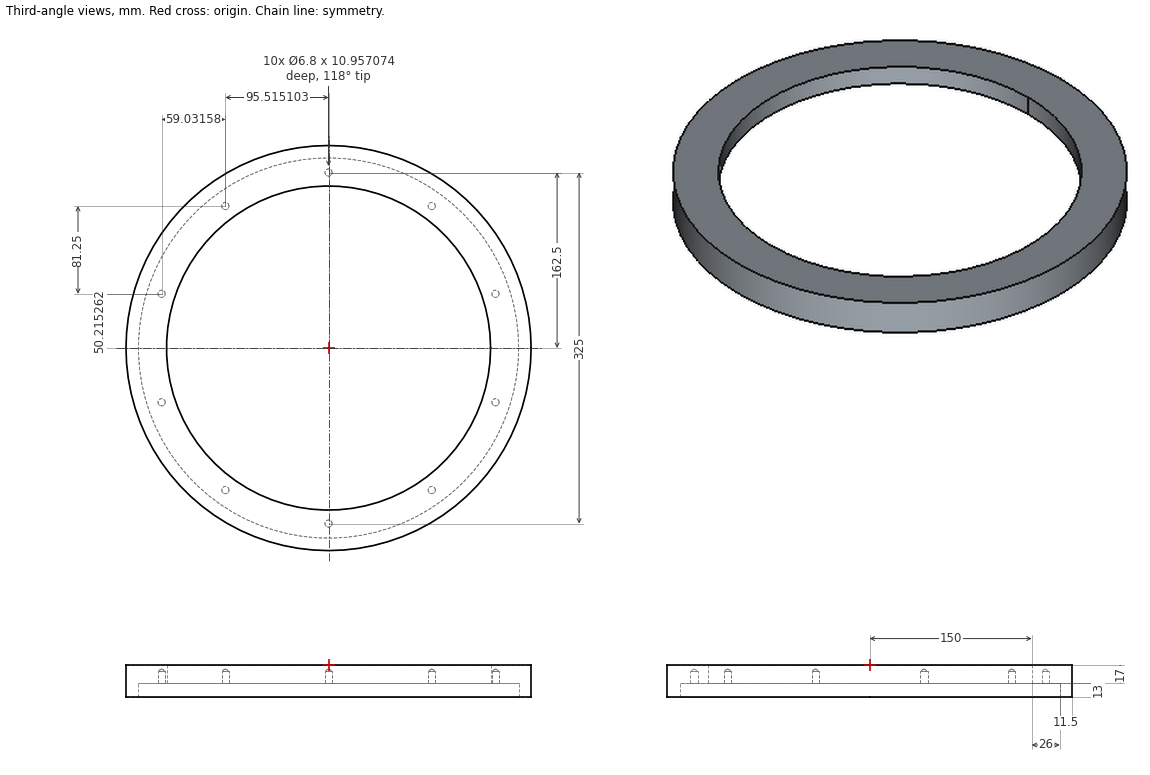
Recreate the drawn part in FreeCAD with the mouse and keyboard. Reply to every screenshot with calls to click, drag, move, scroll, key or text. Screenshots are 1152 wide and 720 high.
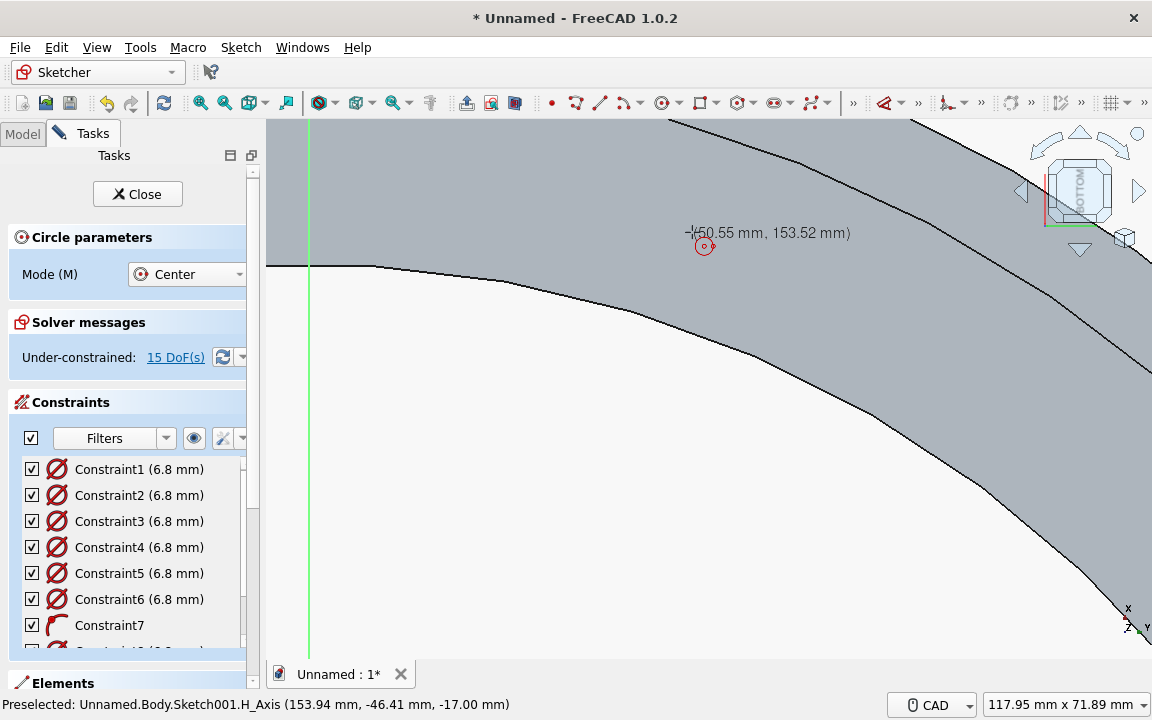
scroll(692, 232, down, 10)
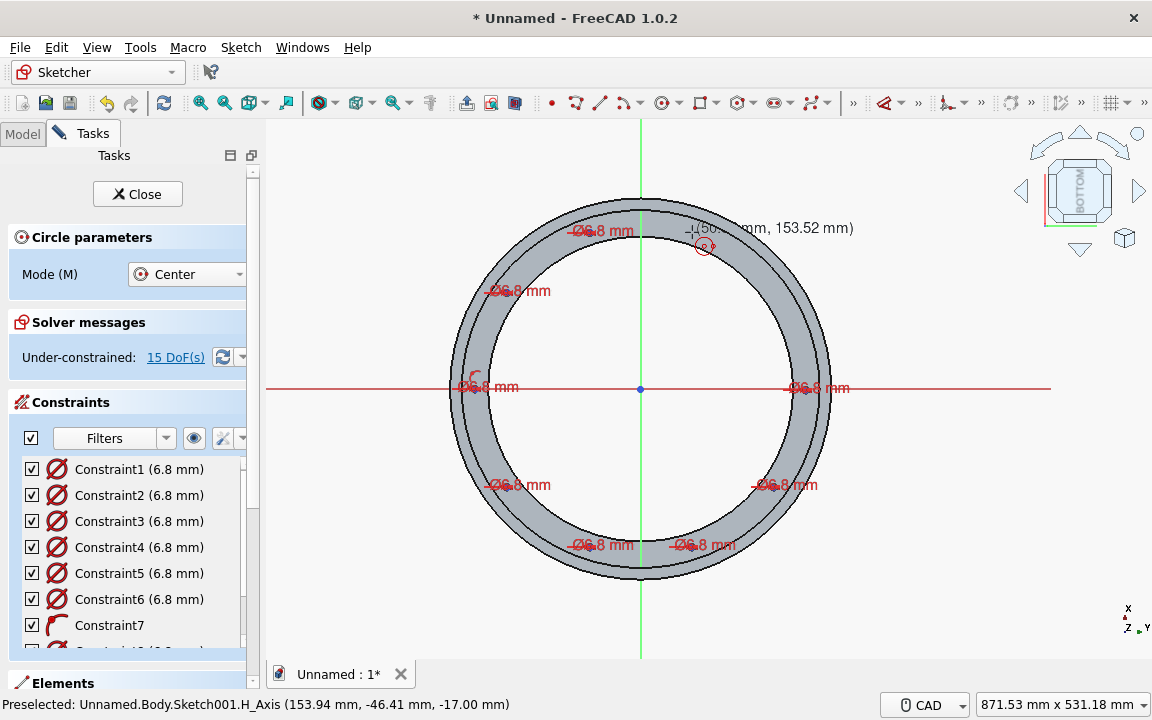
click(692, 232)
move(694, 230)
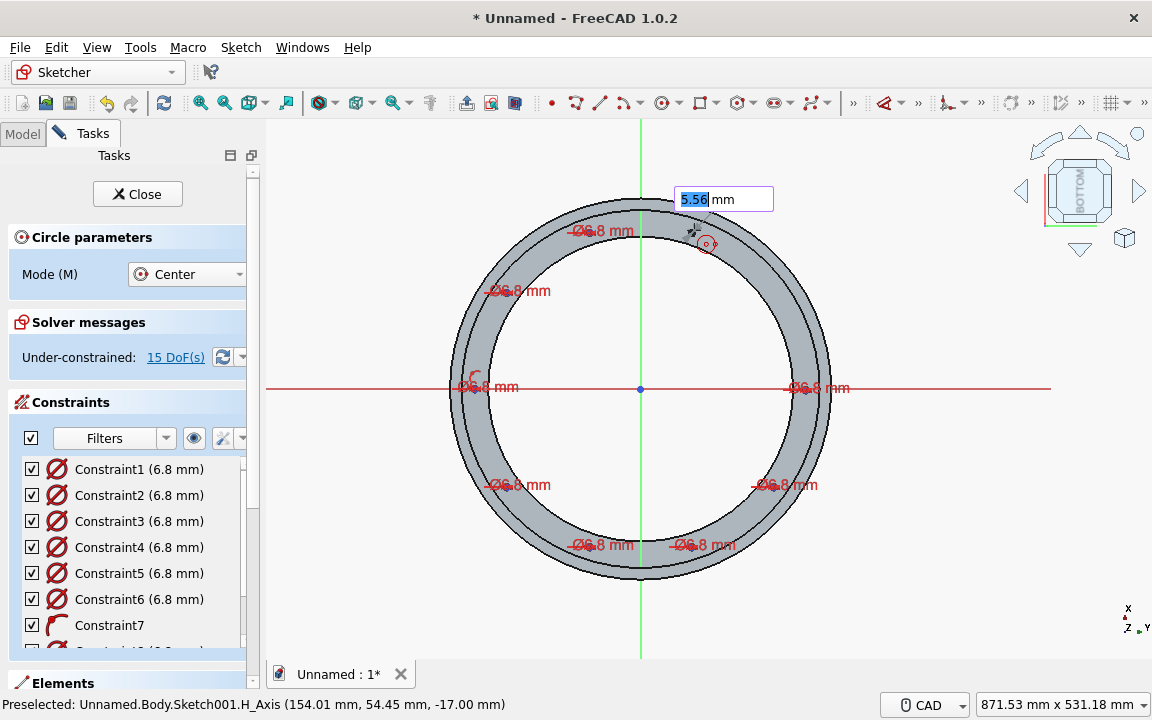
text(6.8)
key(Return)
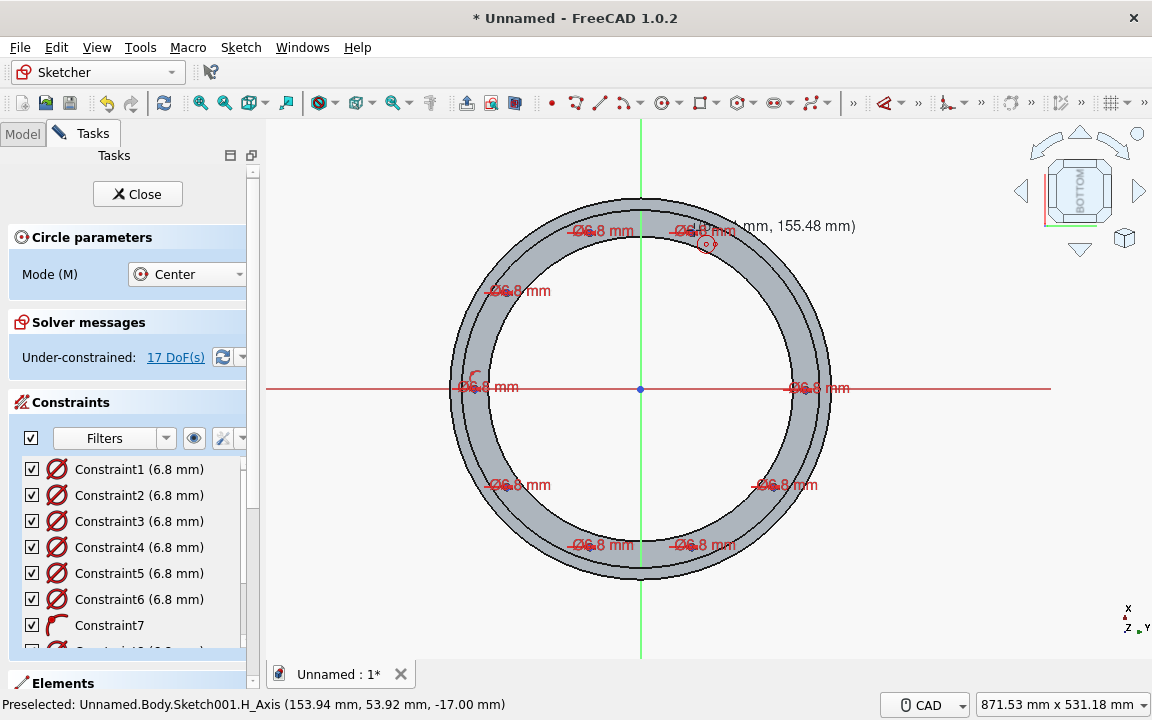
scroll(774, 292, up, 10)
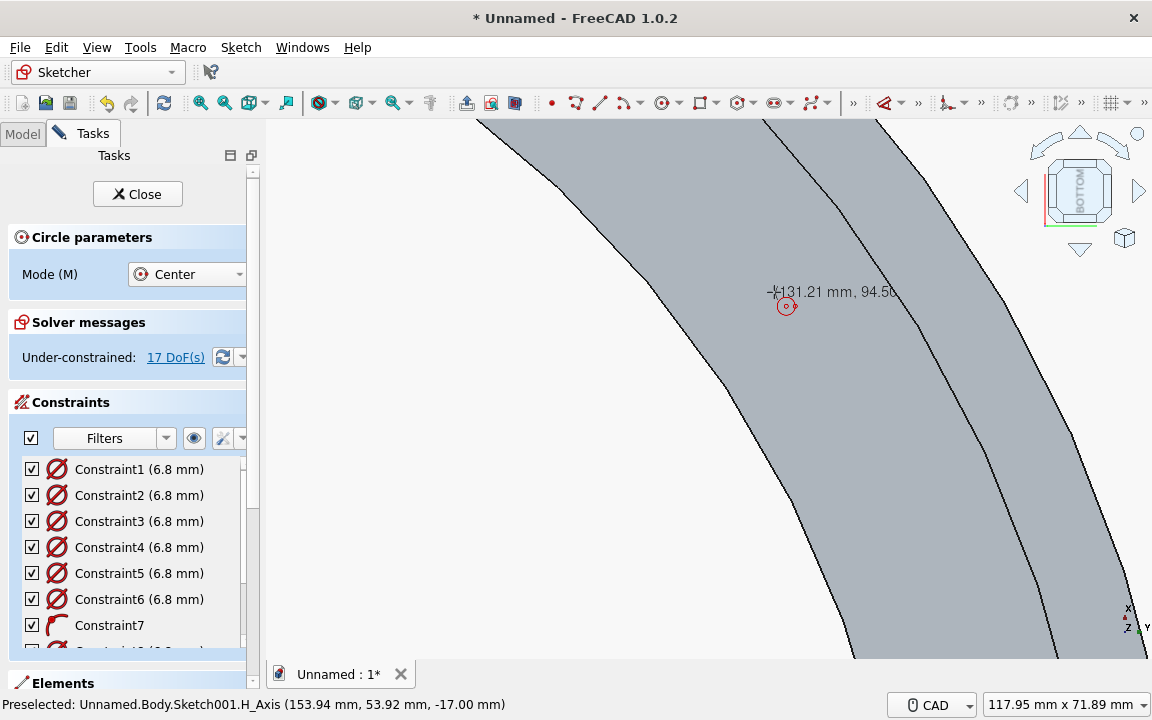
scroll(774, 292, down, 10)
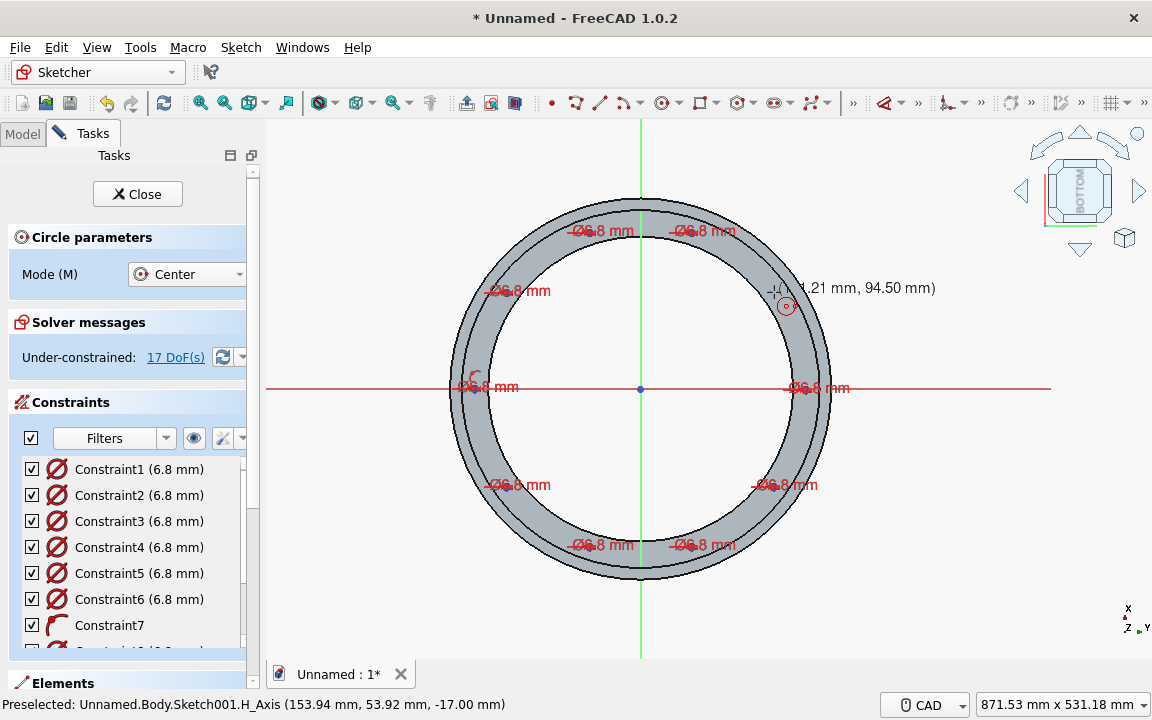
click(774, 292)
move(777, 290)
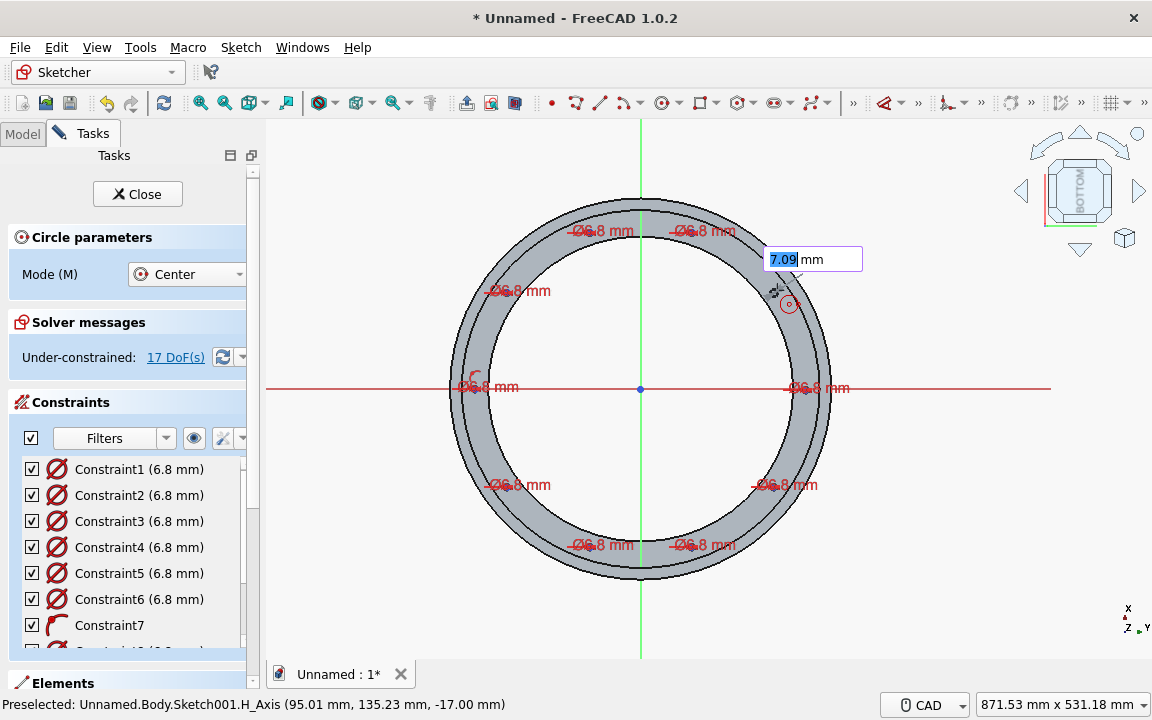
text(6.8)
key(Return)
key(Escape)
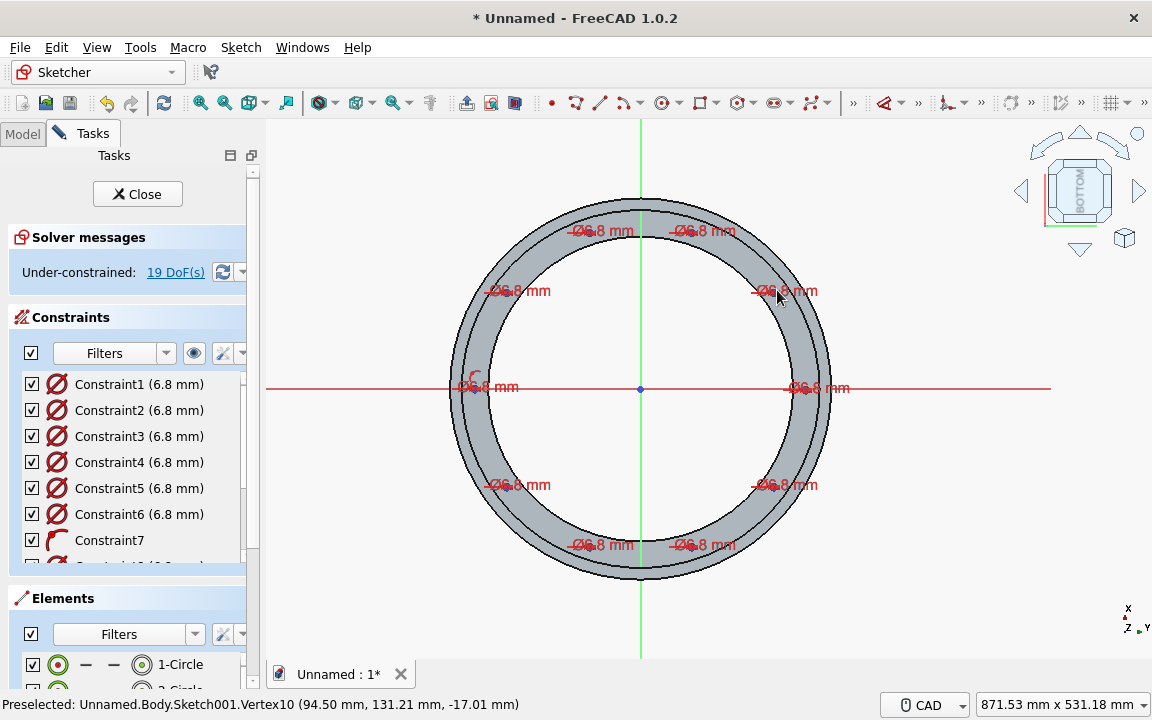
click(806, 390)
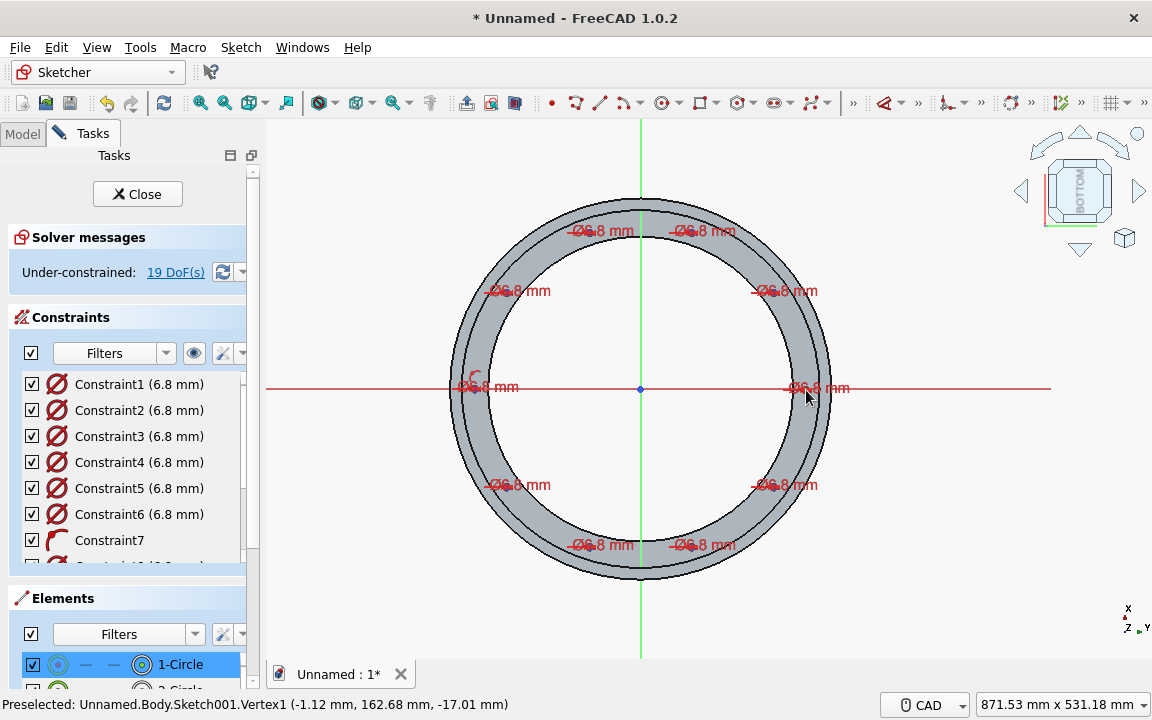
click(344, 389)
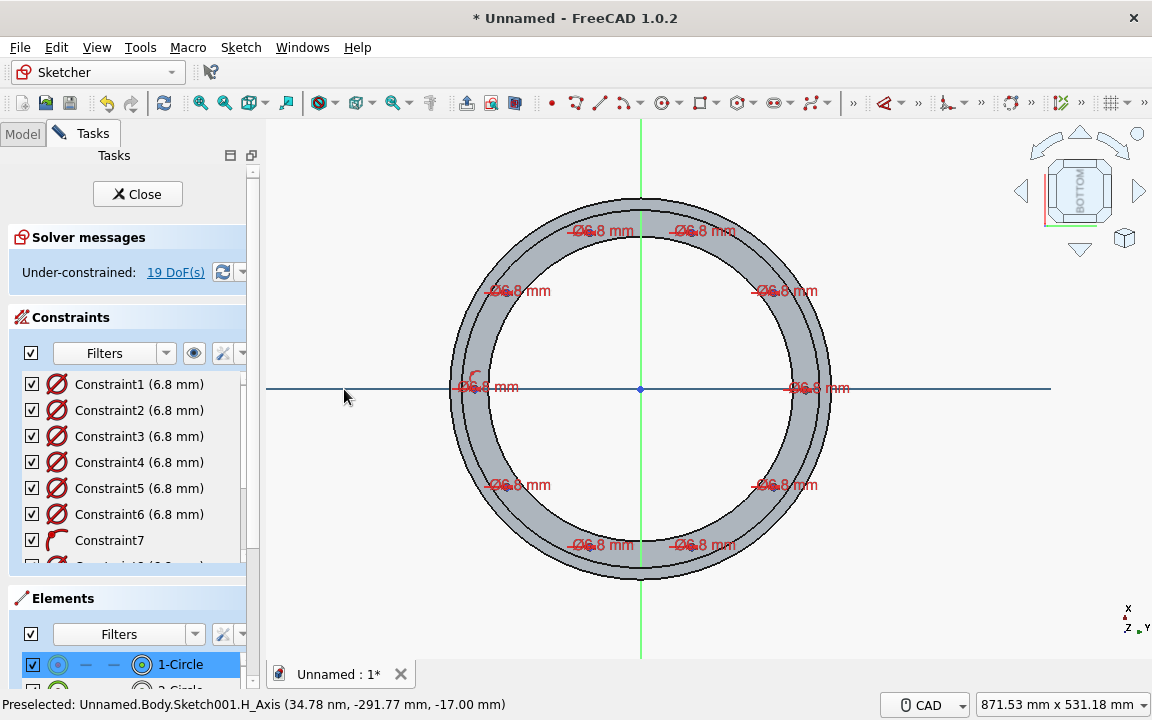
key(c)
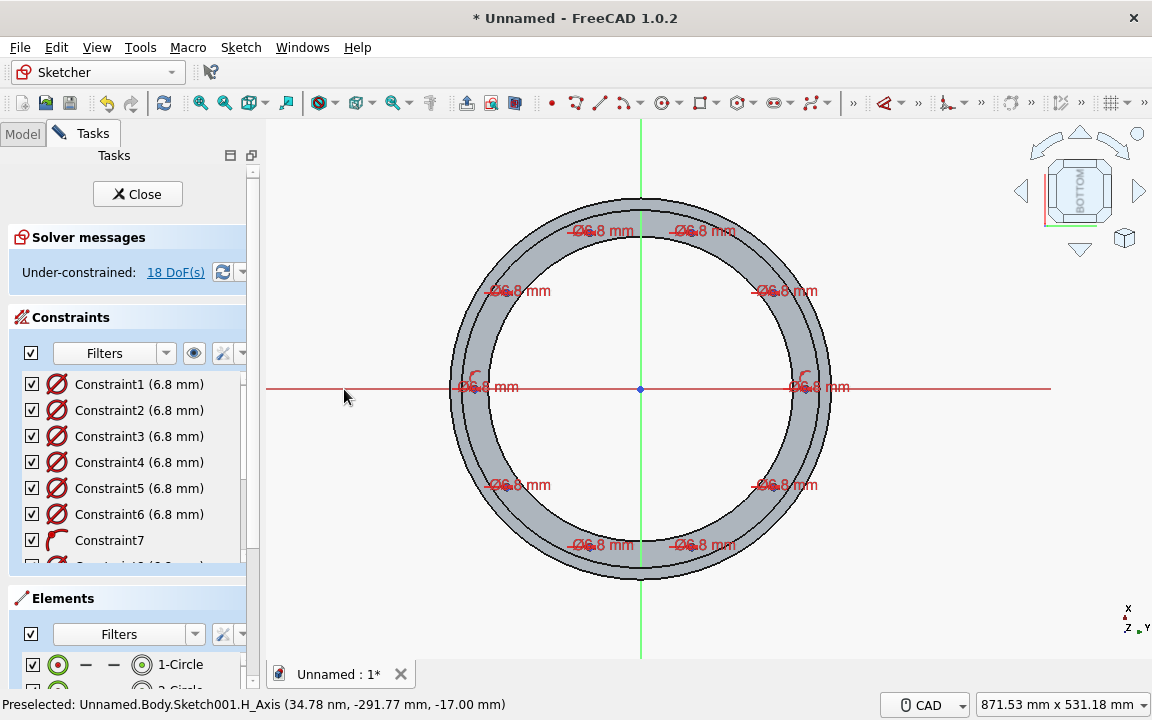
click(692, 547)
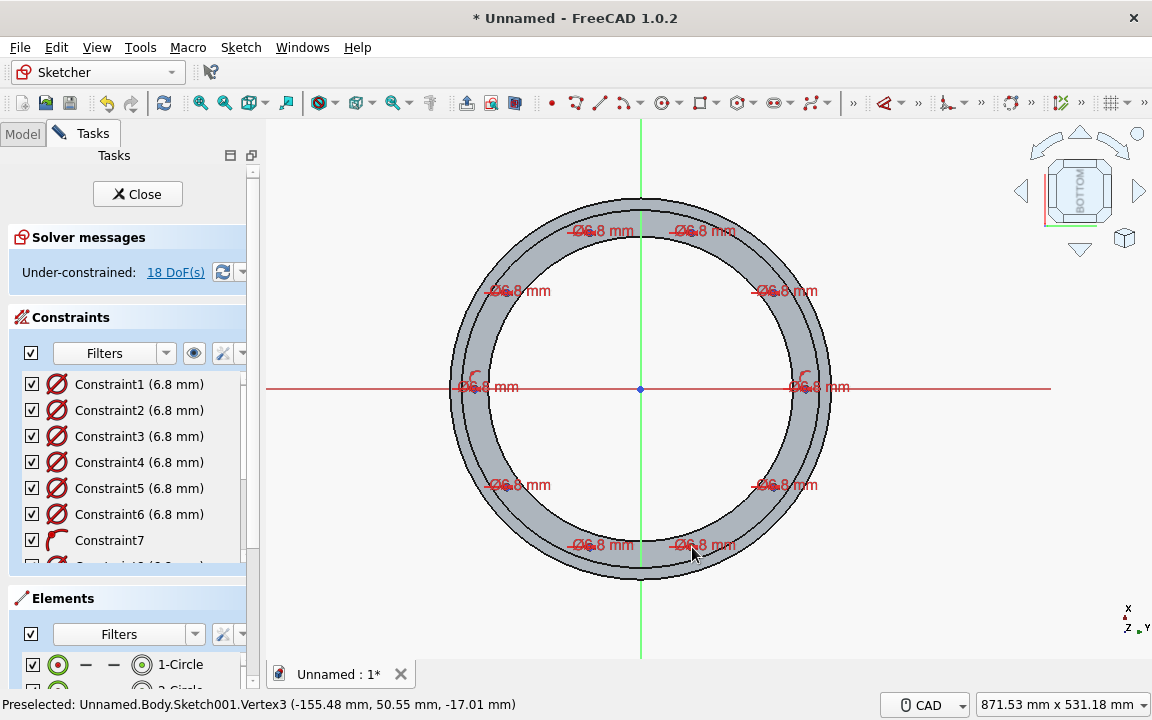
click(590, 547)